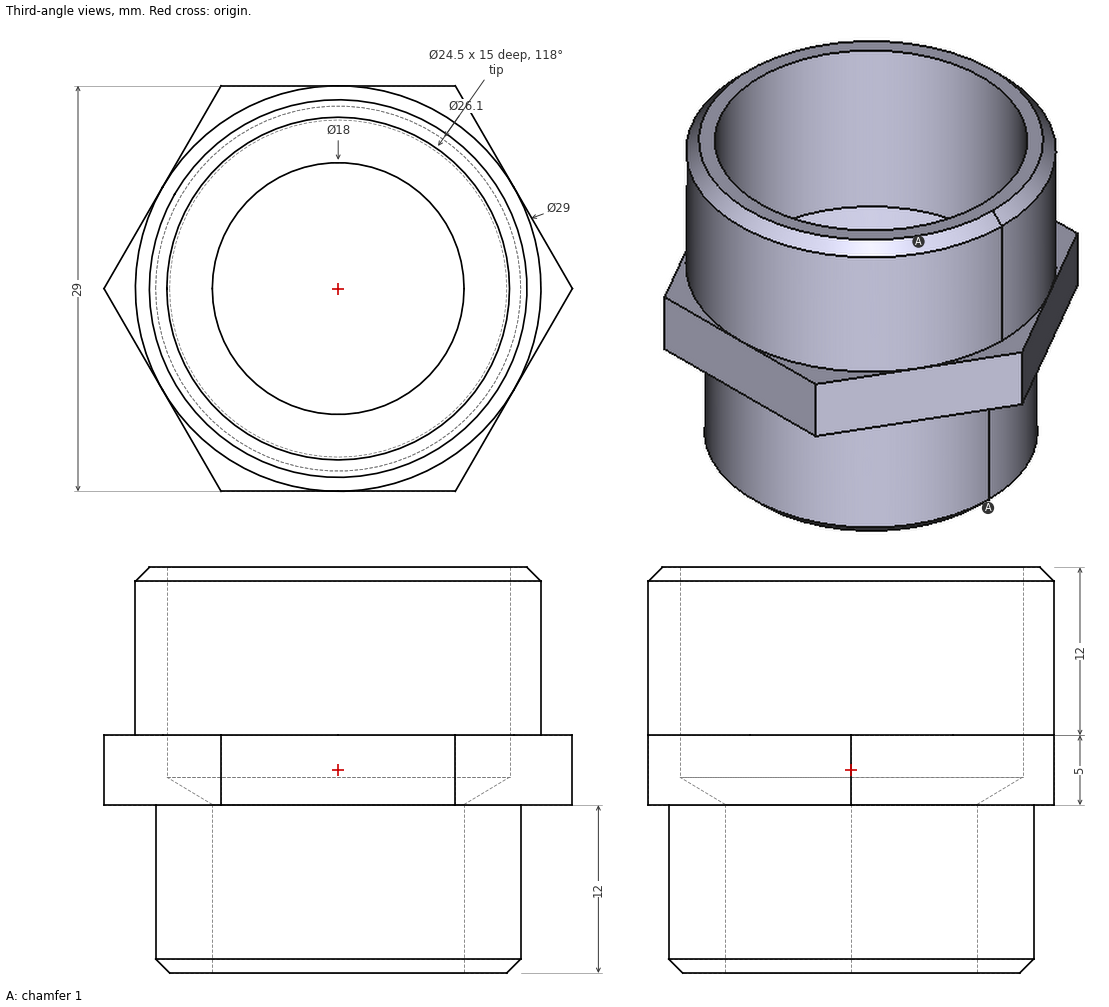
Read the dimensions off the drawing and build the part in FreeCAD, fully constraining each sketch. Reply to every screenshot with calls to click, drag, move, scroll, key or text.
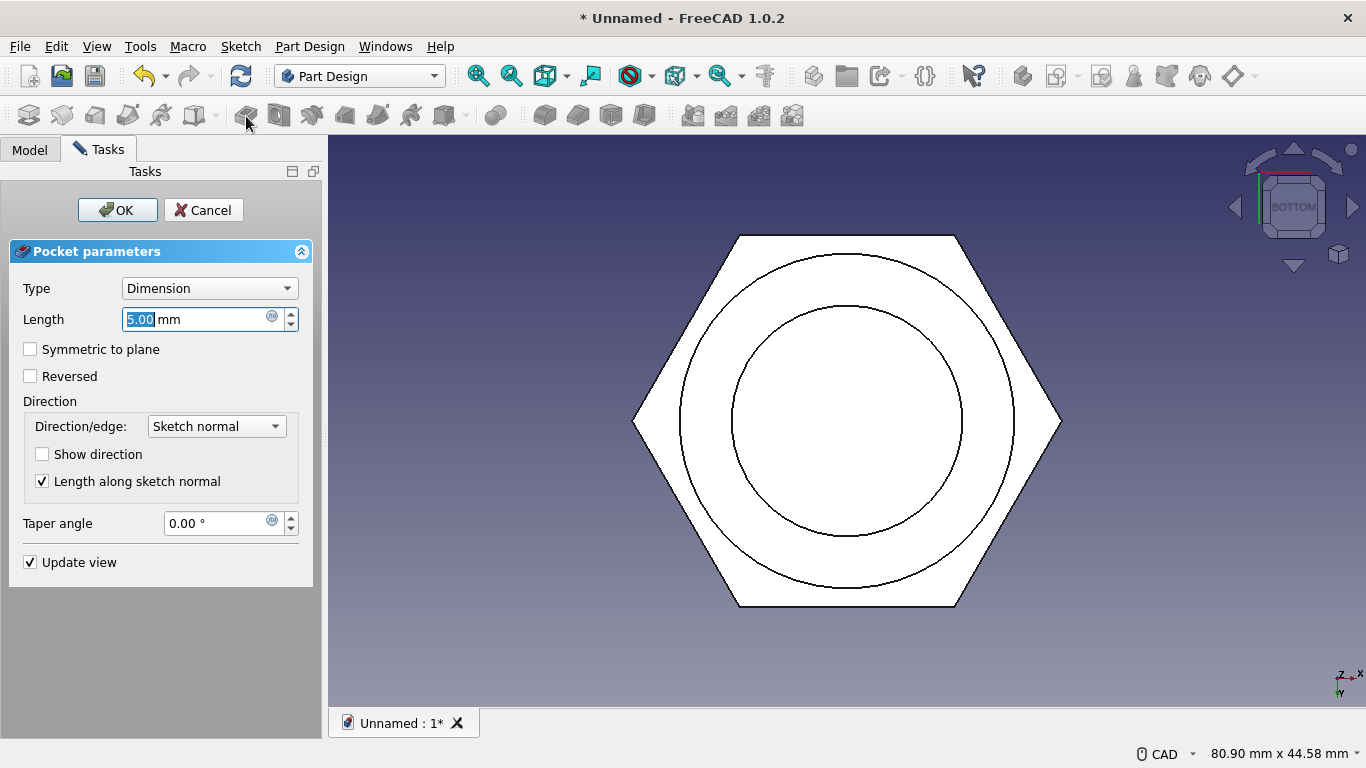
click(210, 288)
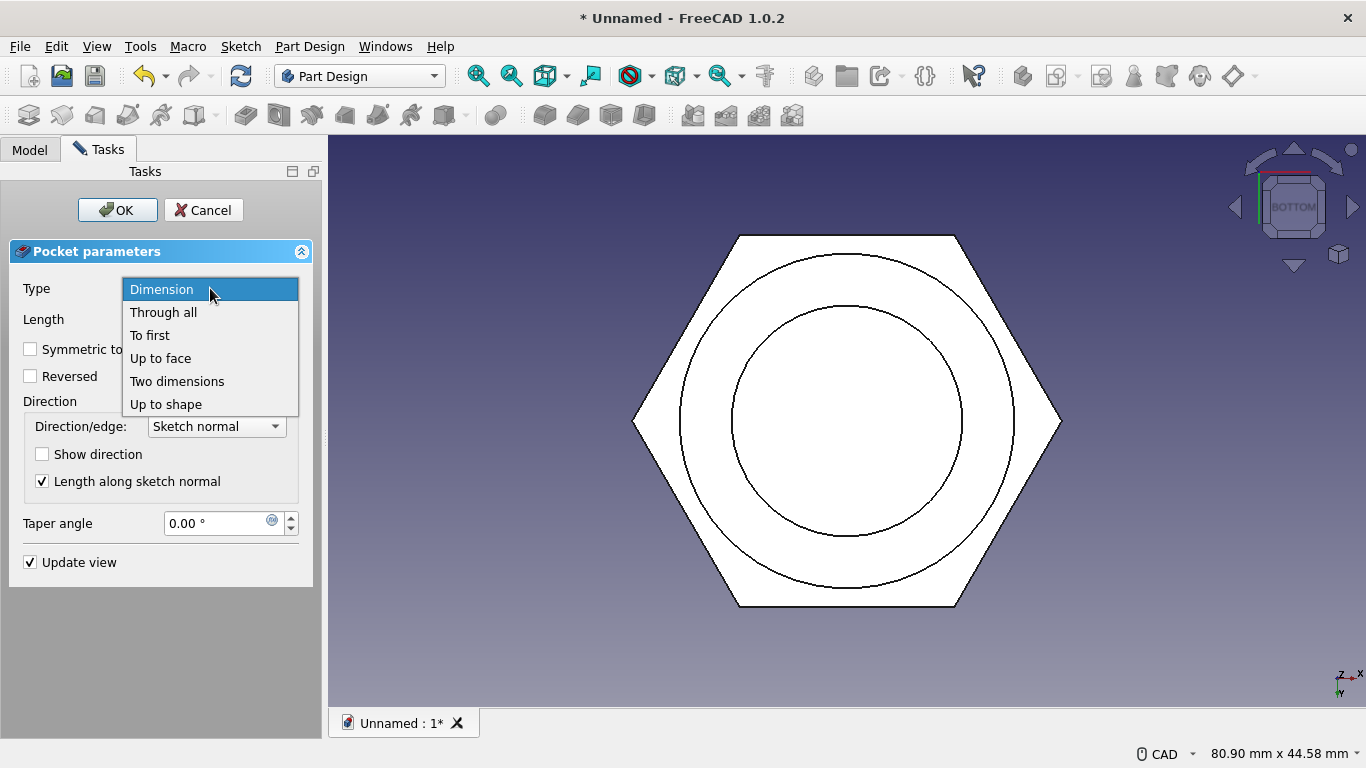
click(208, 336)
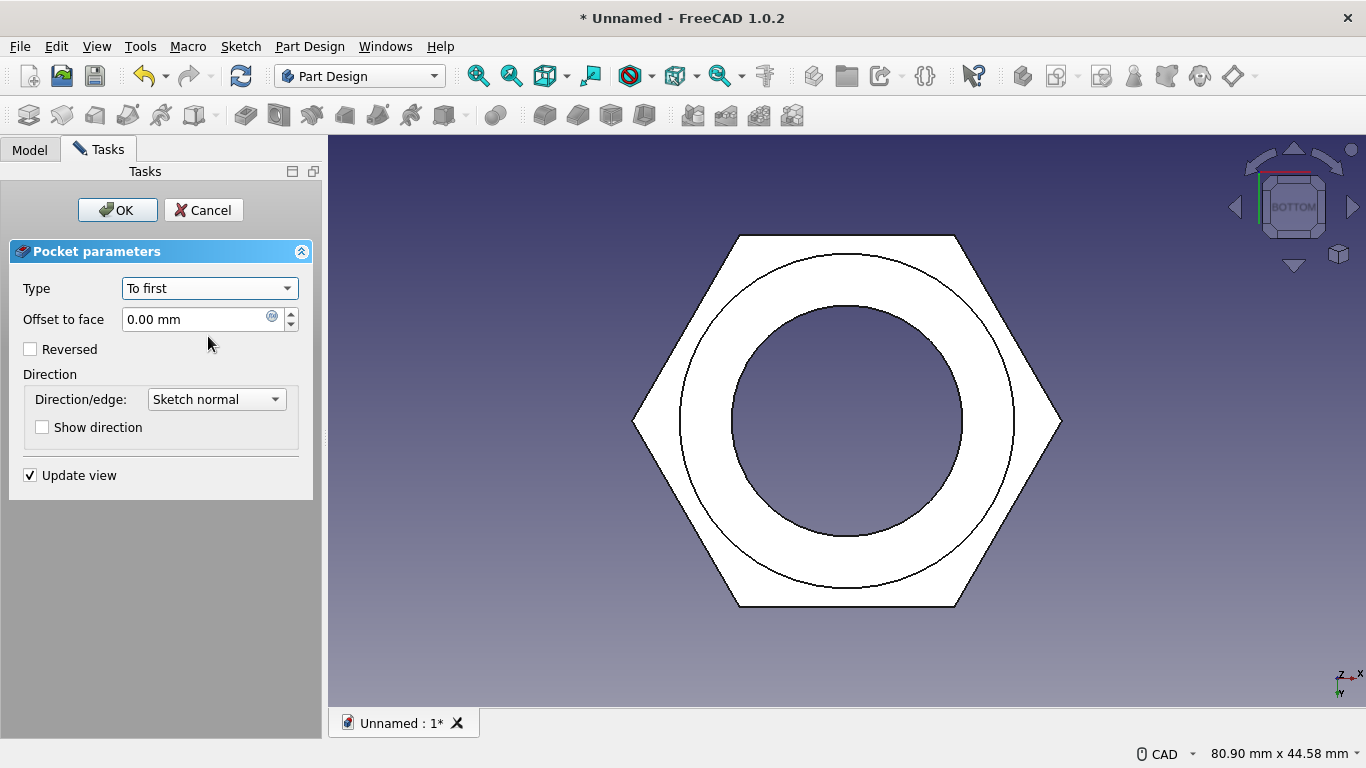
click(118, 210)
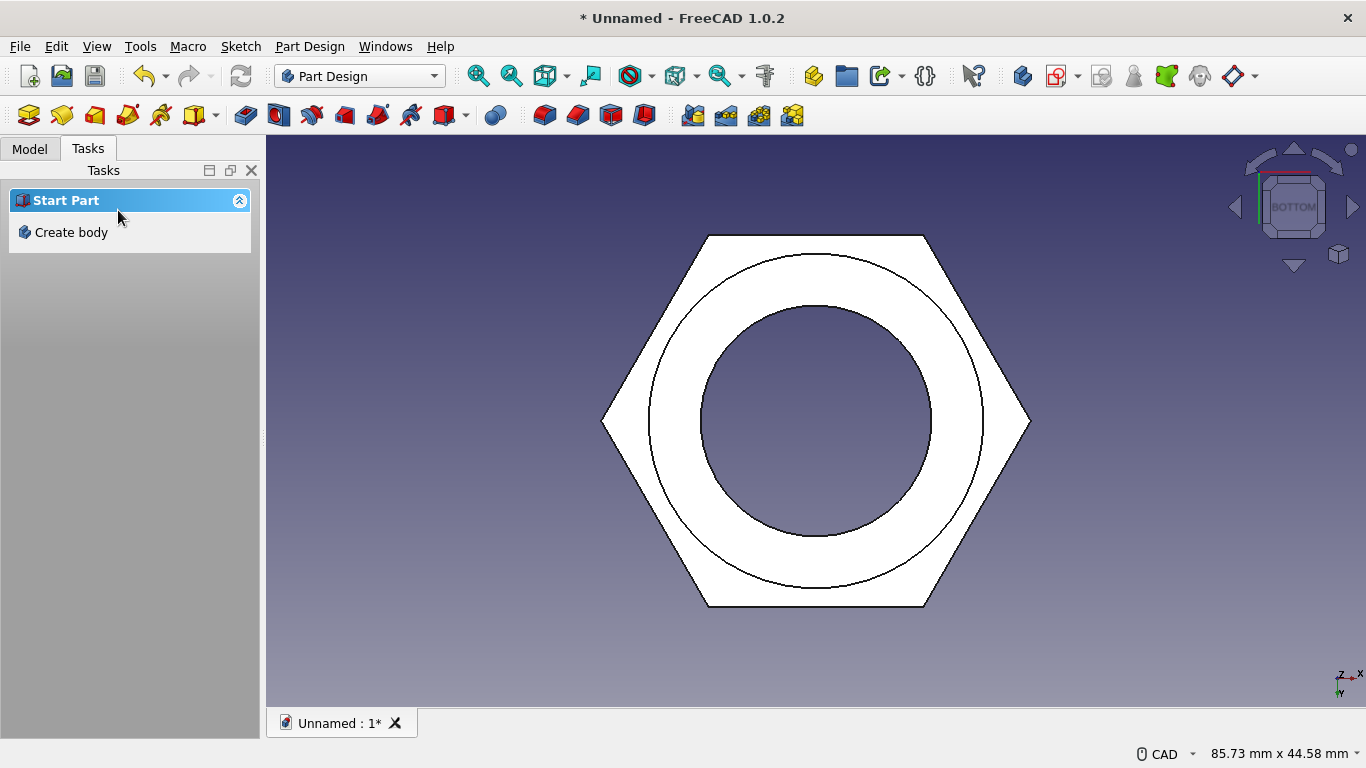
key(0)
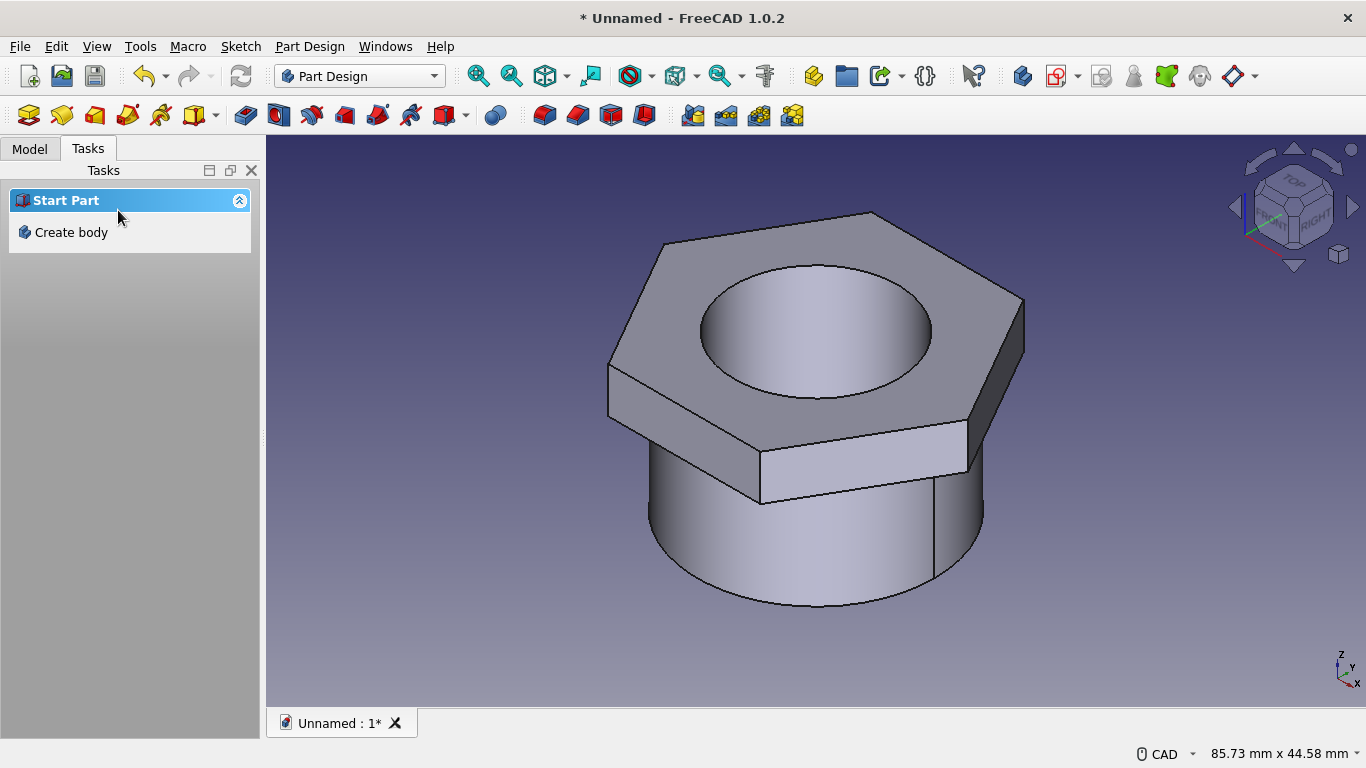
click(804, 237)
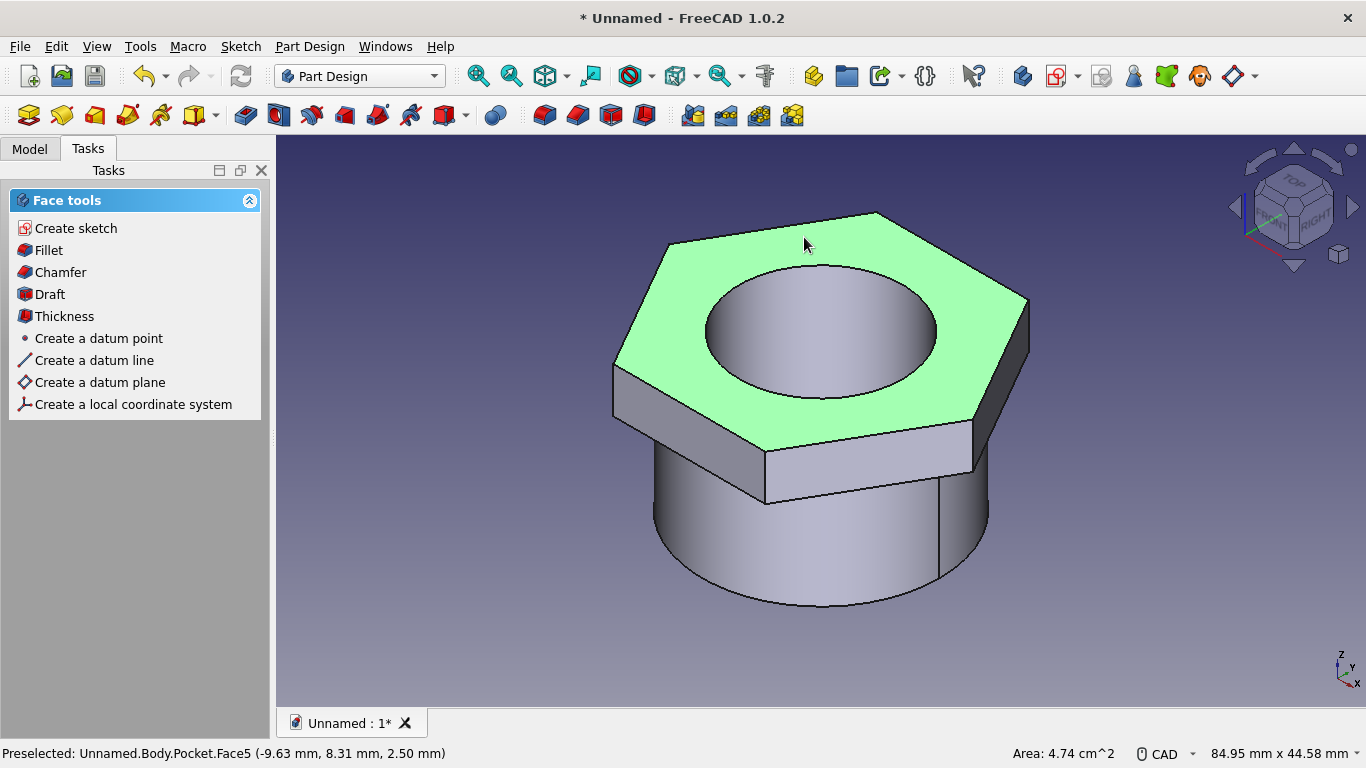
click(1056, 76)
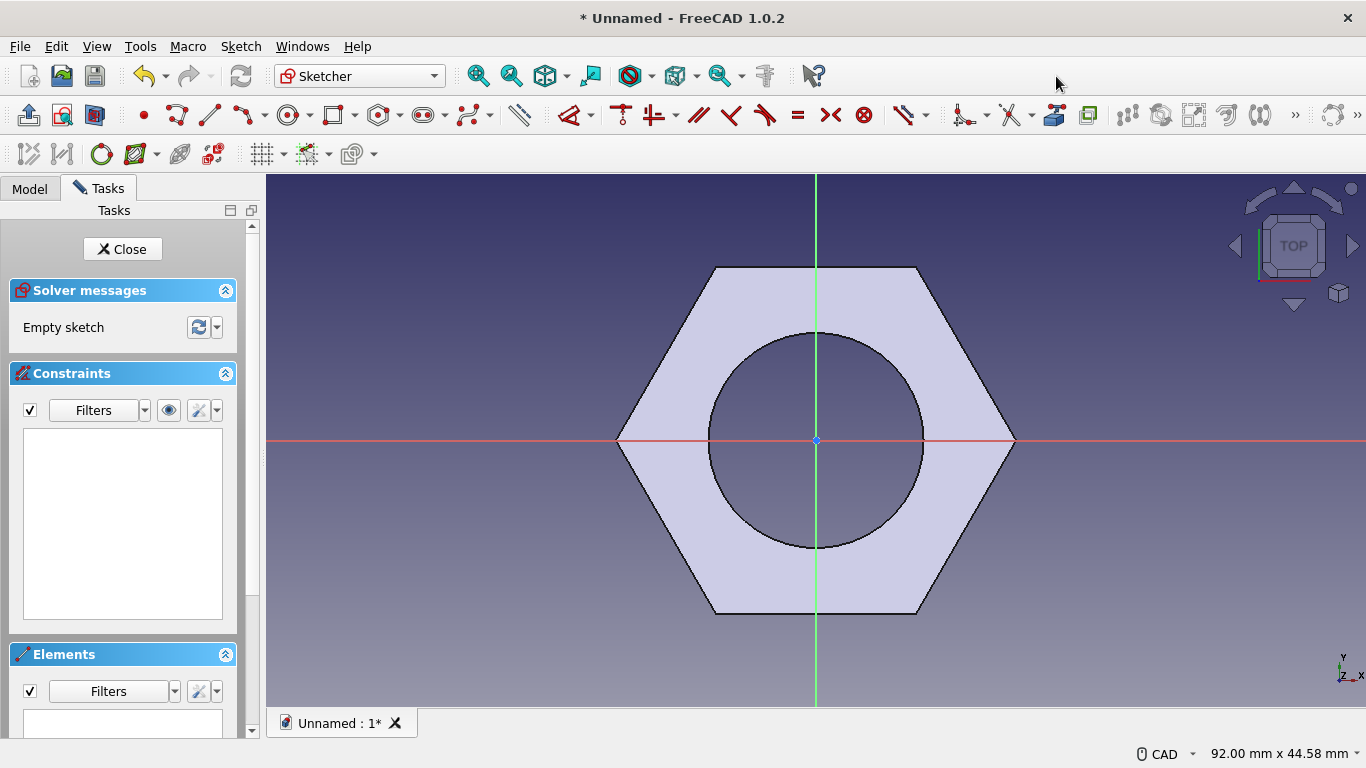
click(288, 116)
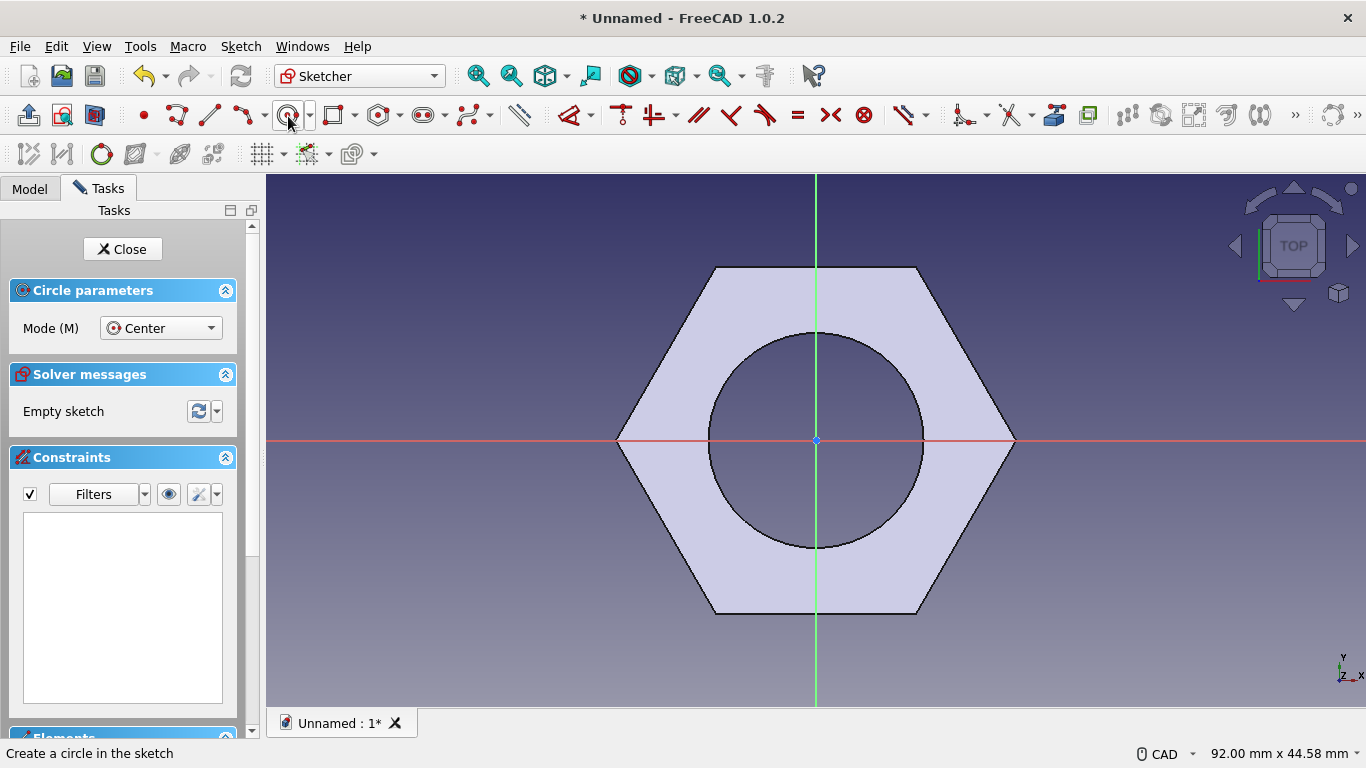
click(816, 440)
move(939, 318)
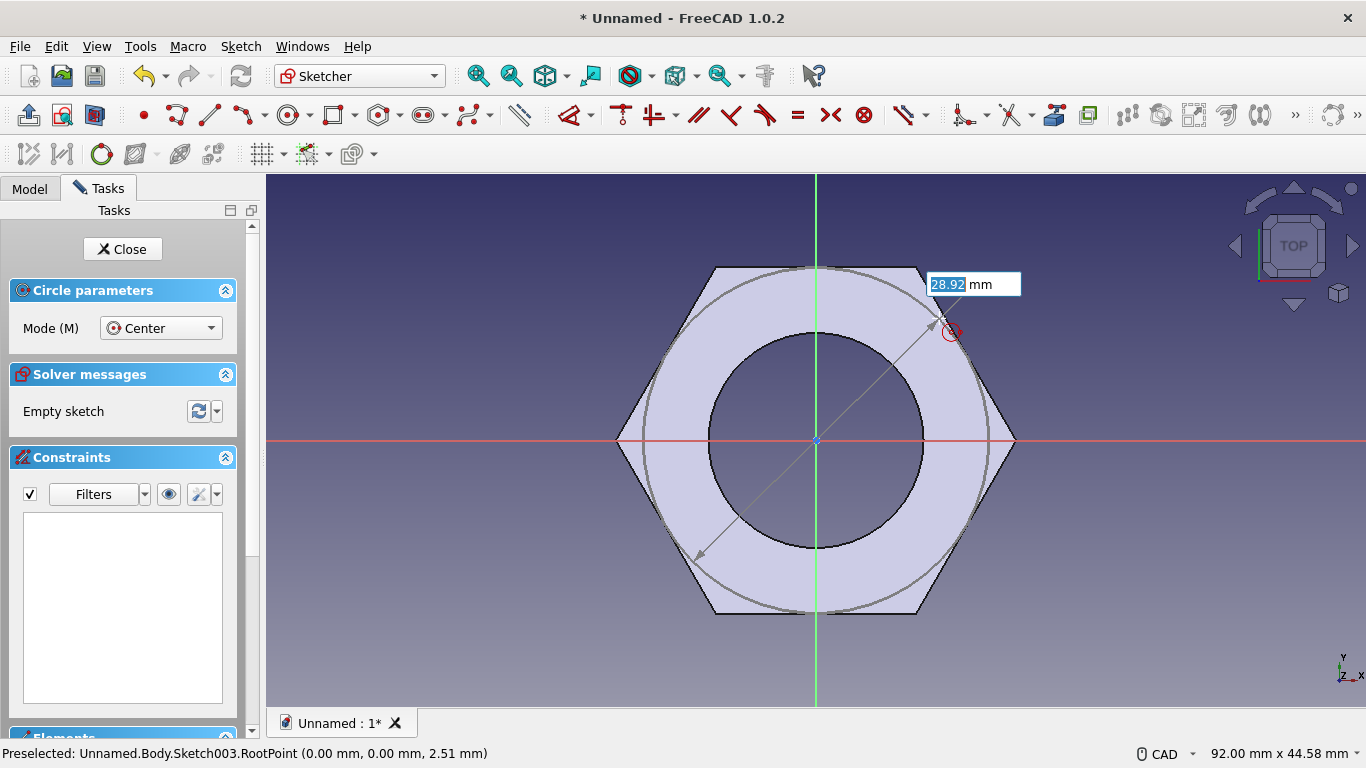
text(29)
key(Return)